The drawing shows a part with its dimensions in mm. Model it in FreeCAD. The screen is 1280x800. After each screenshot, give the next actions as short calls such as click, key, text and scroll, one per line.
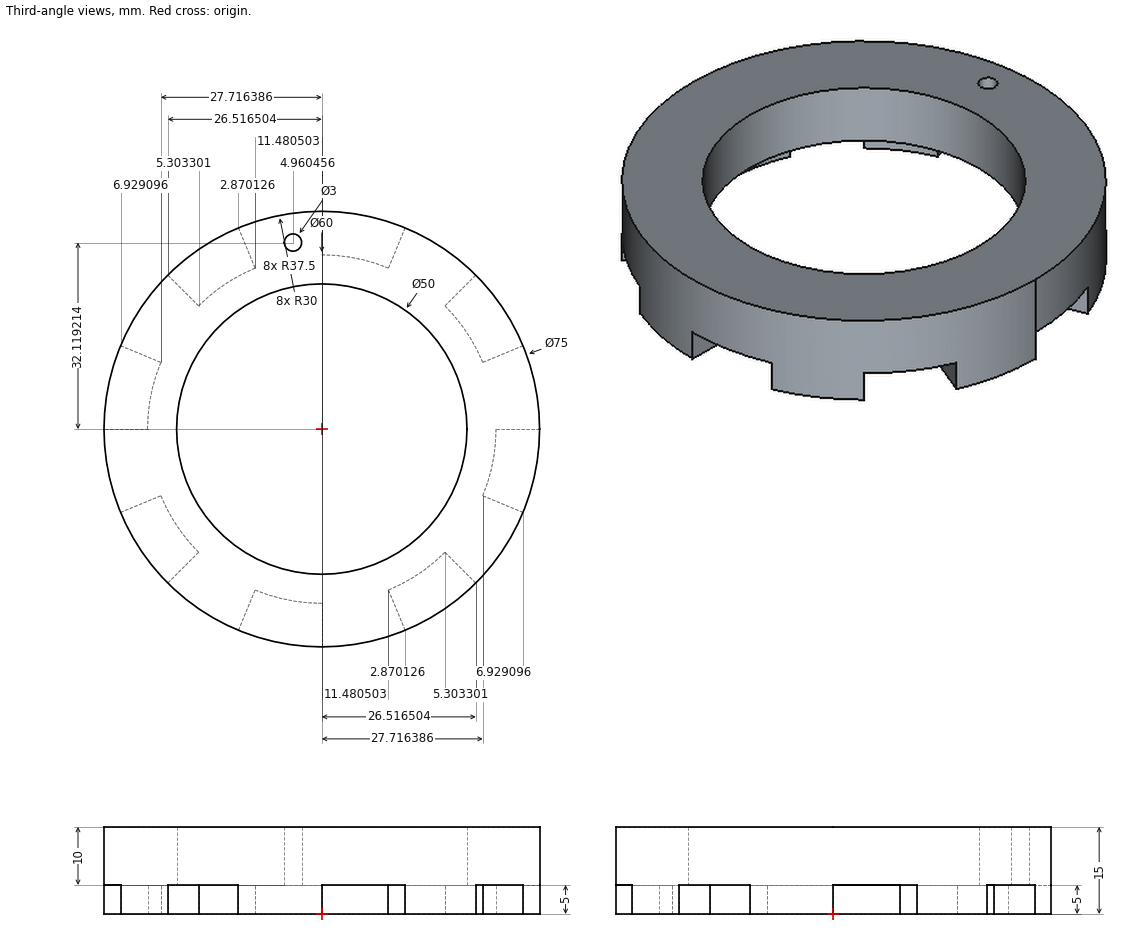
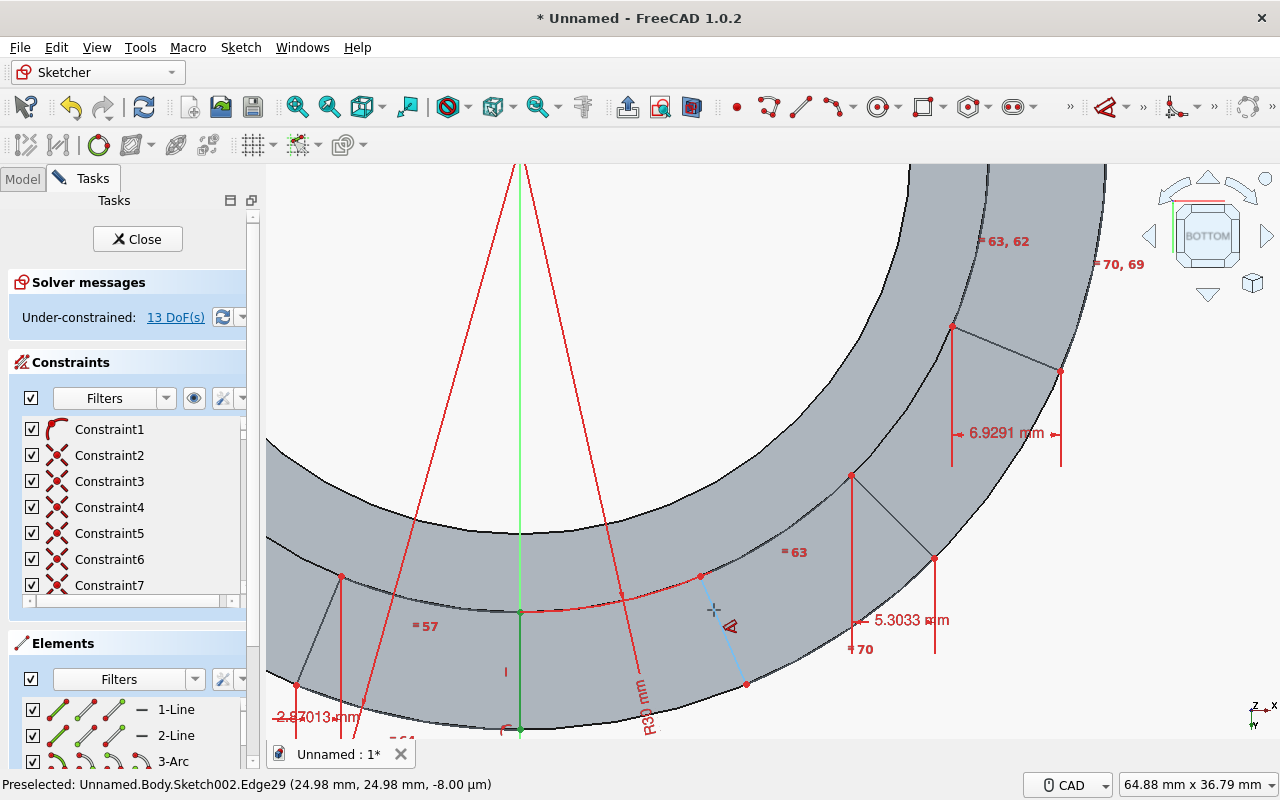
click(714, 609)
click(723, 543)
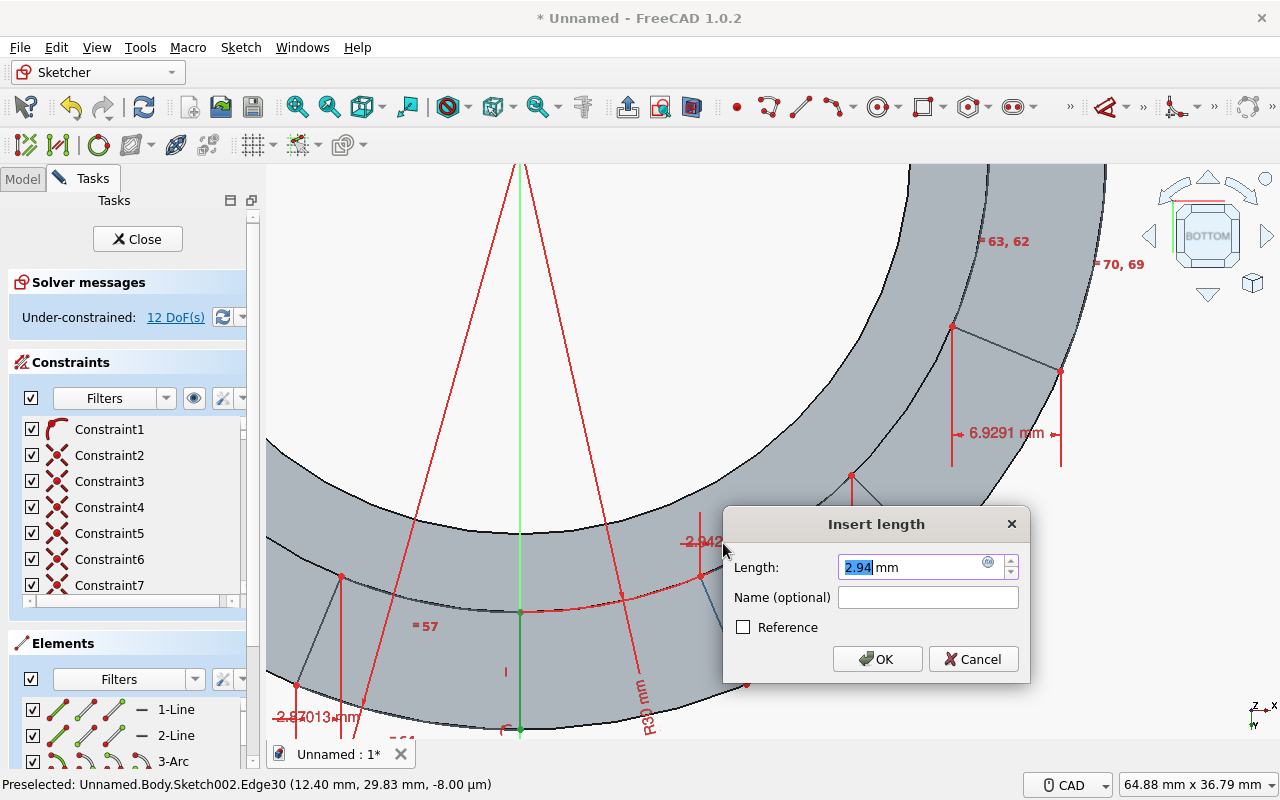
text(2.870126)
key(Return)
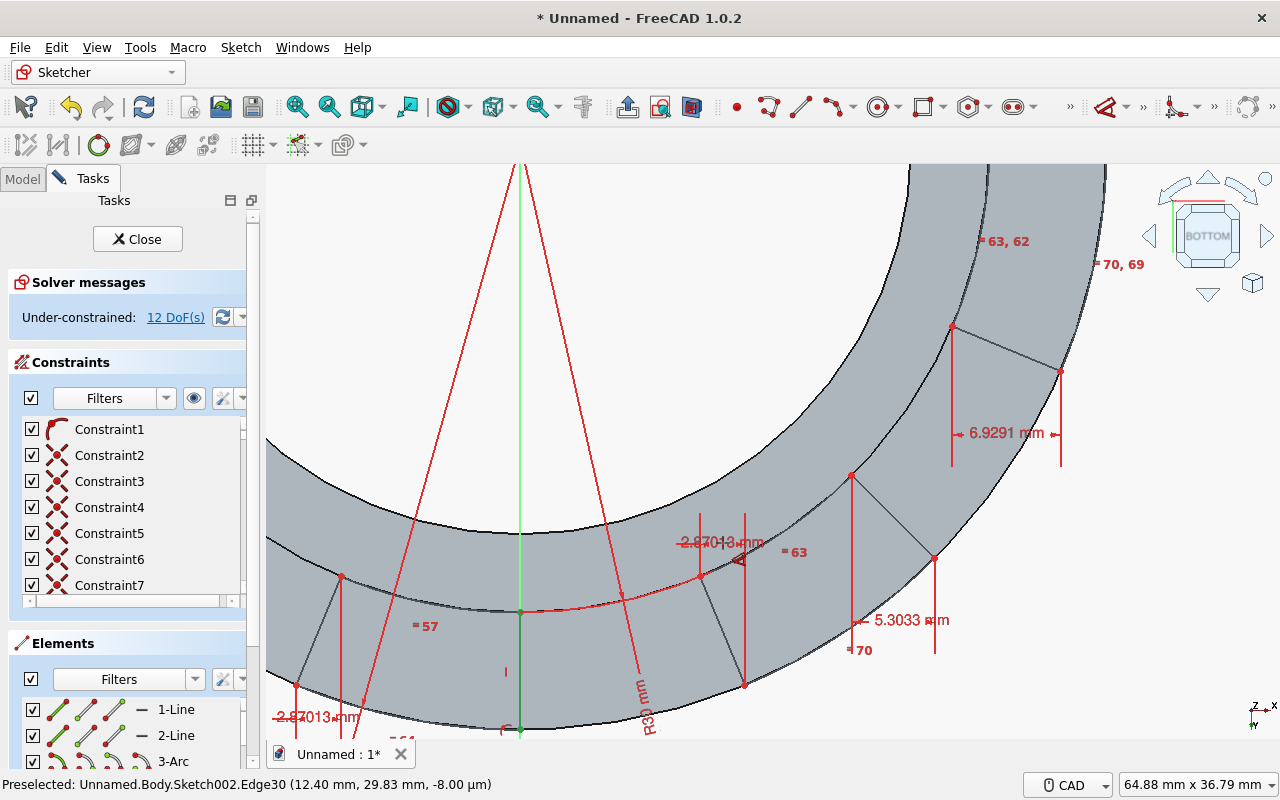
click(341, 577)
click(389, 611)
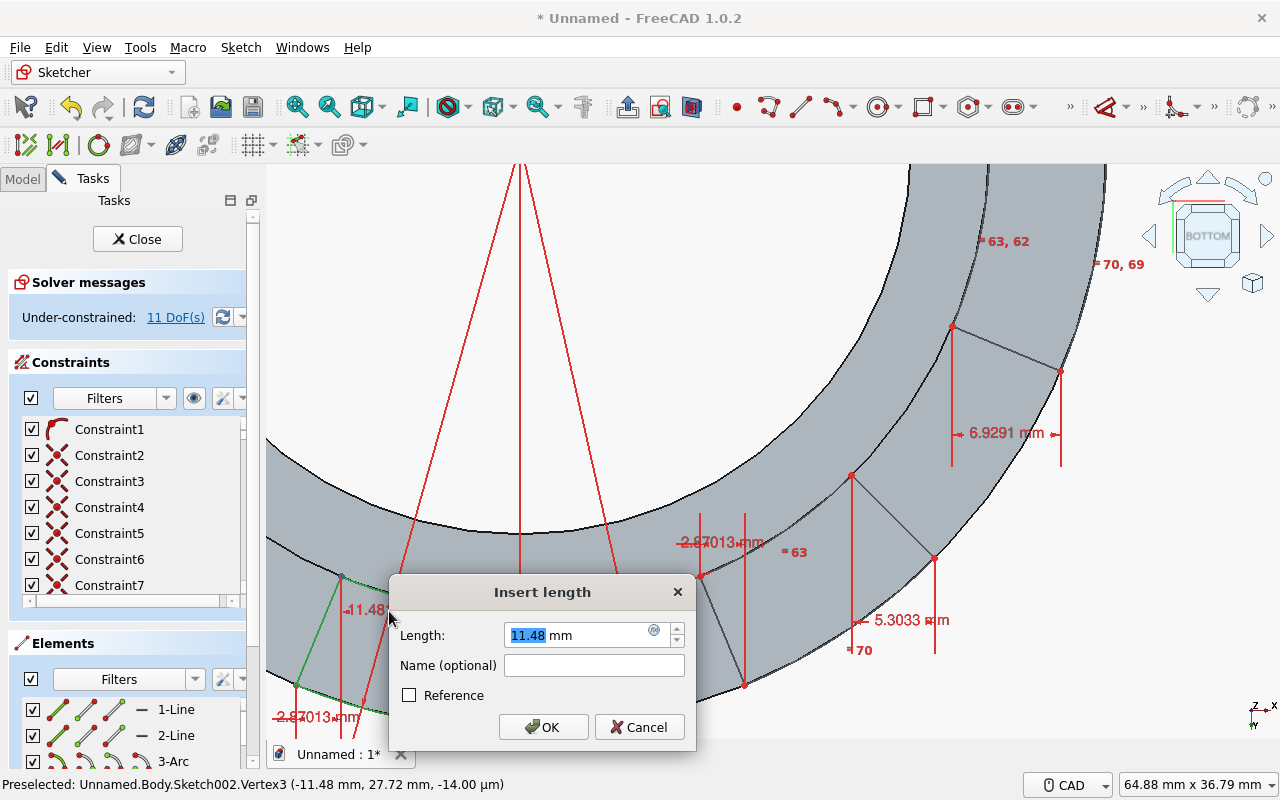
text(11.480503)
key(Return)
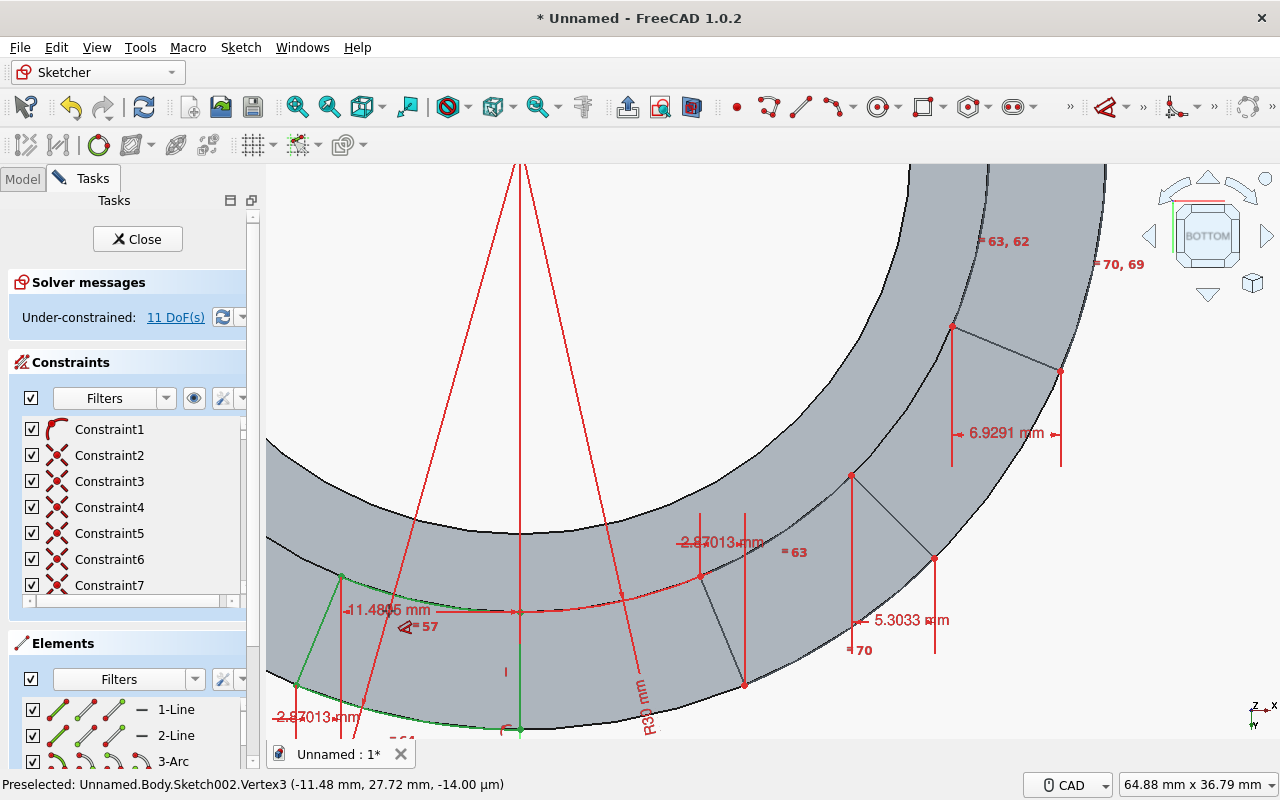
scroll(784, 584, down, 6)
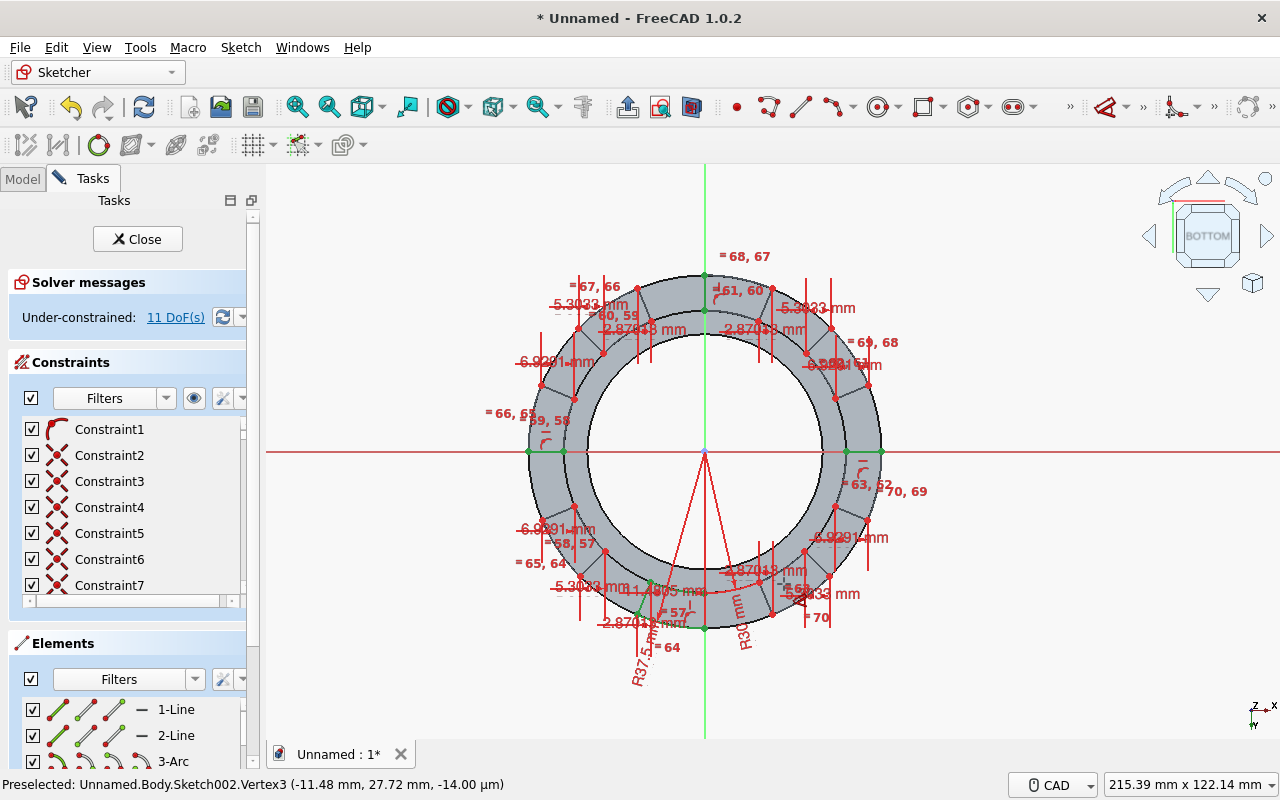
click(580, 577)
click(643, 418)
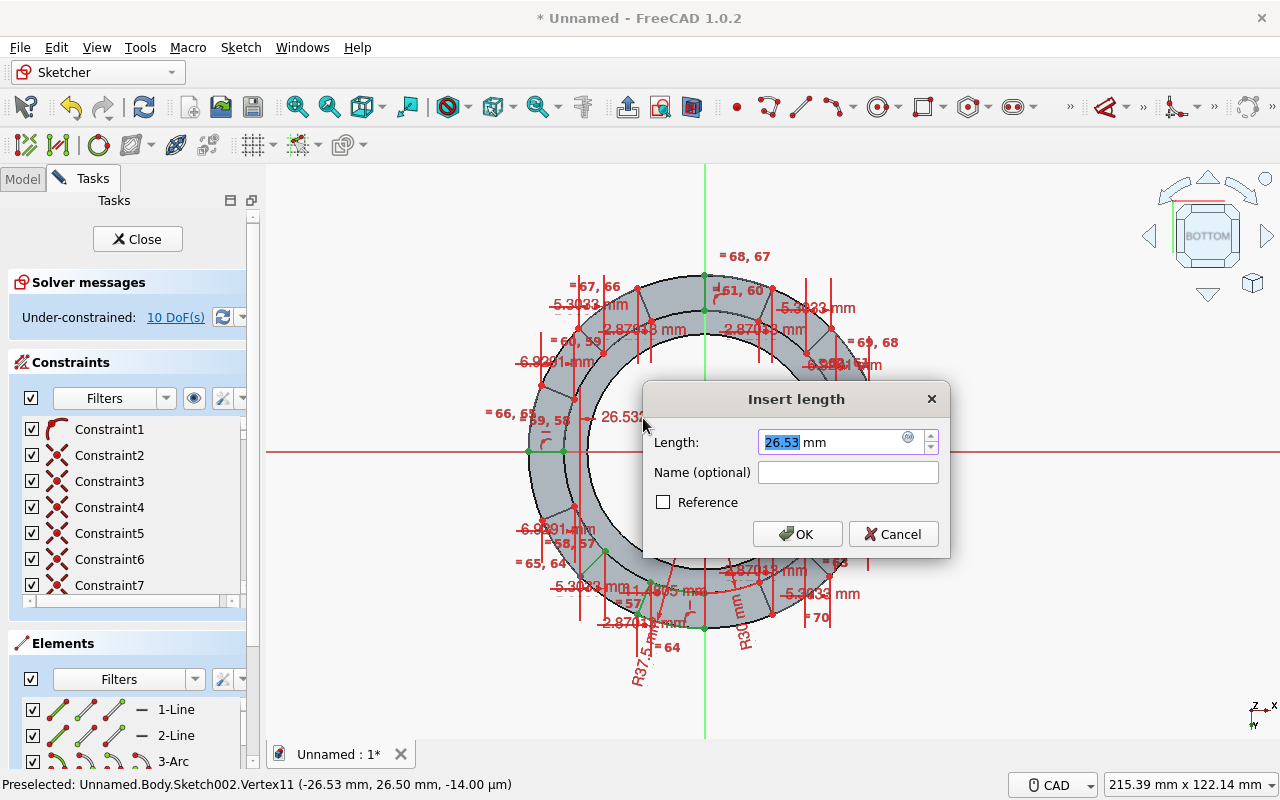
text(26.516504)
key(Return)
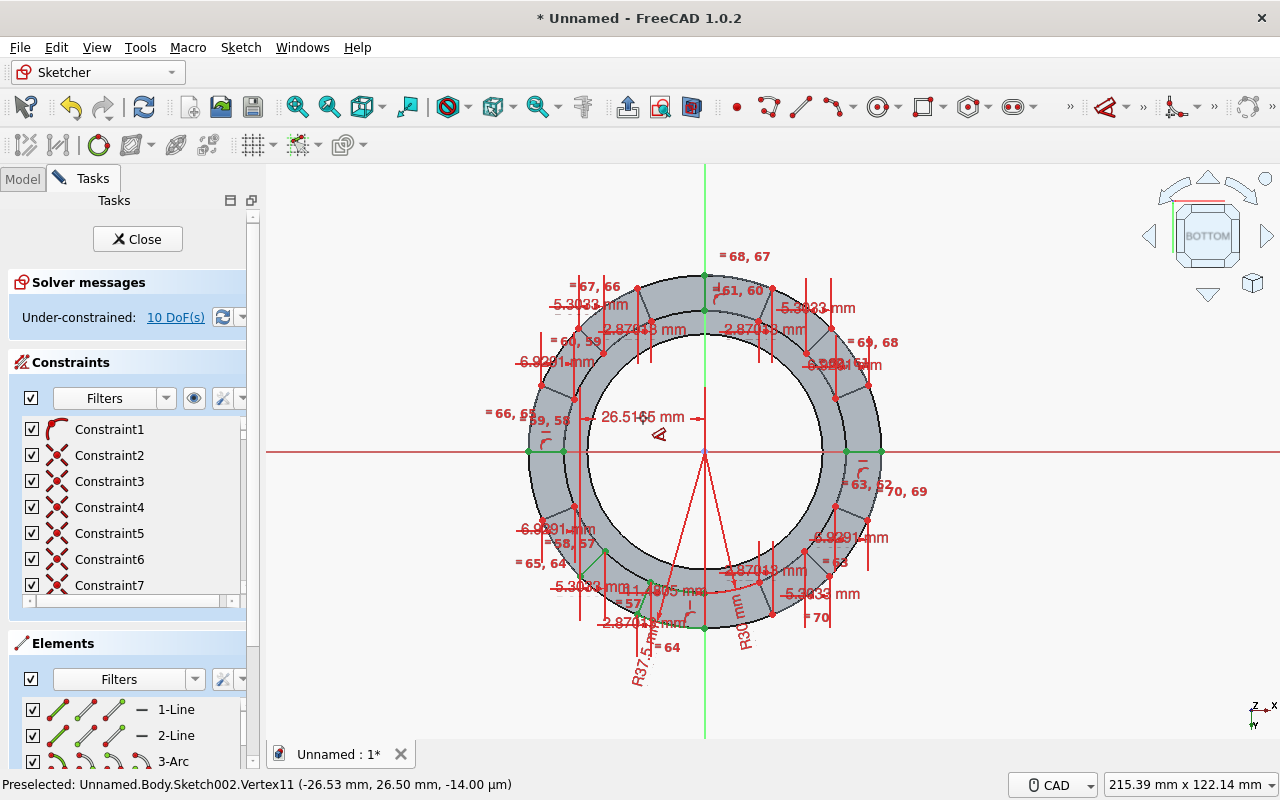
click(575, 507)
click(640, 541)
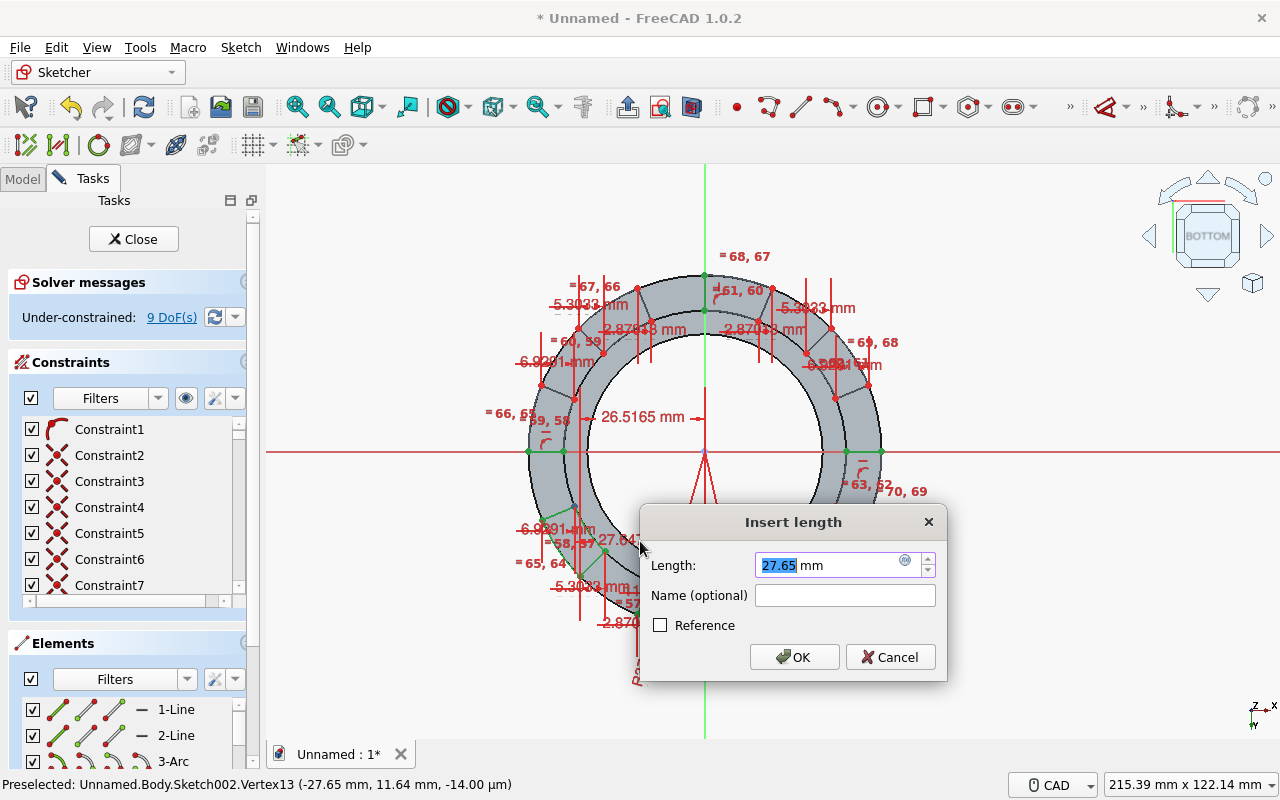
text(27.716386)
key(Return)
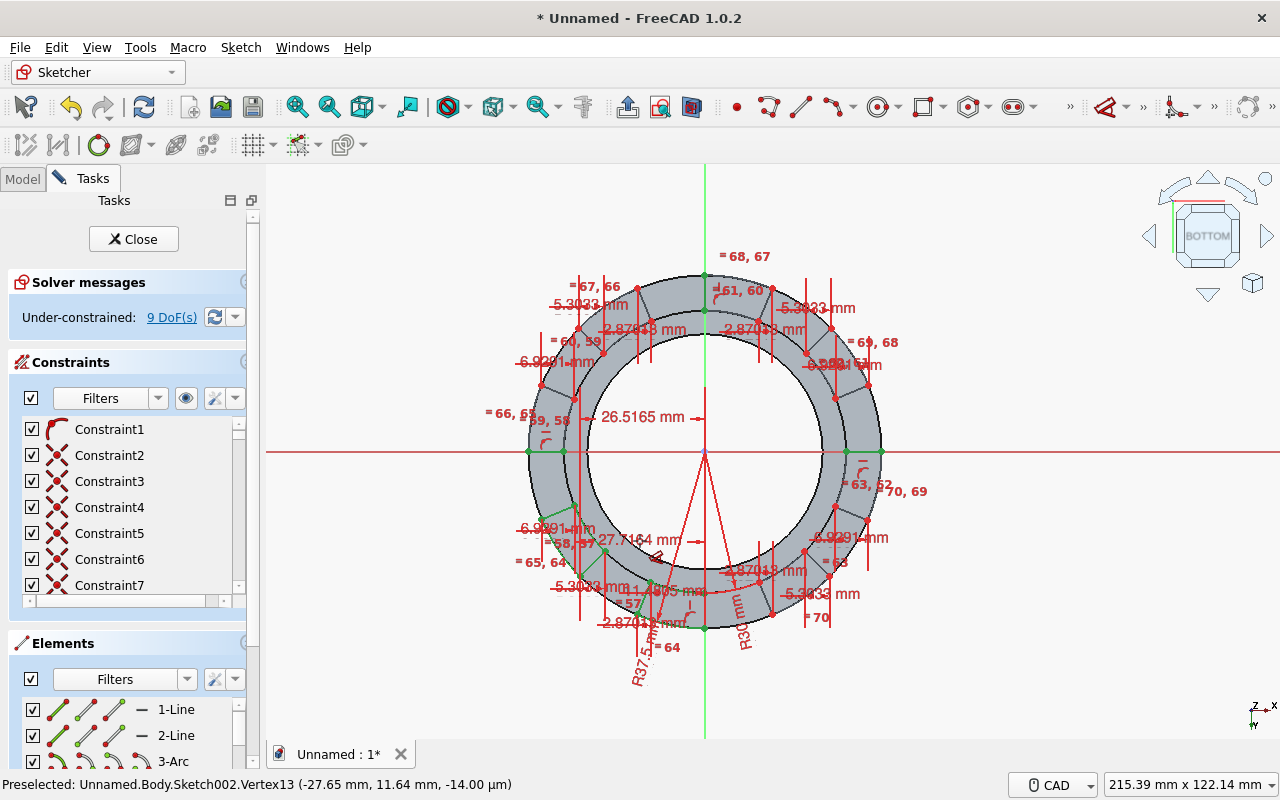
click(574, 399)
click(640, 365)